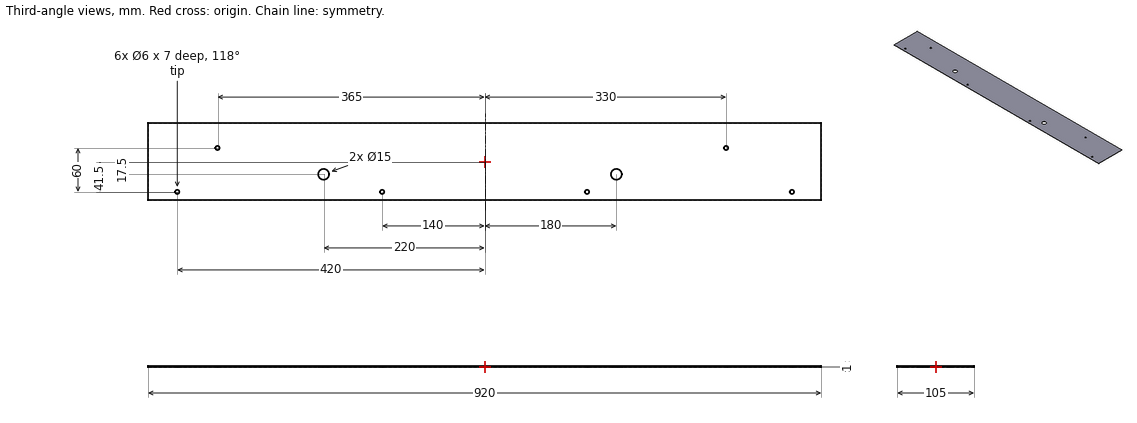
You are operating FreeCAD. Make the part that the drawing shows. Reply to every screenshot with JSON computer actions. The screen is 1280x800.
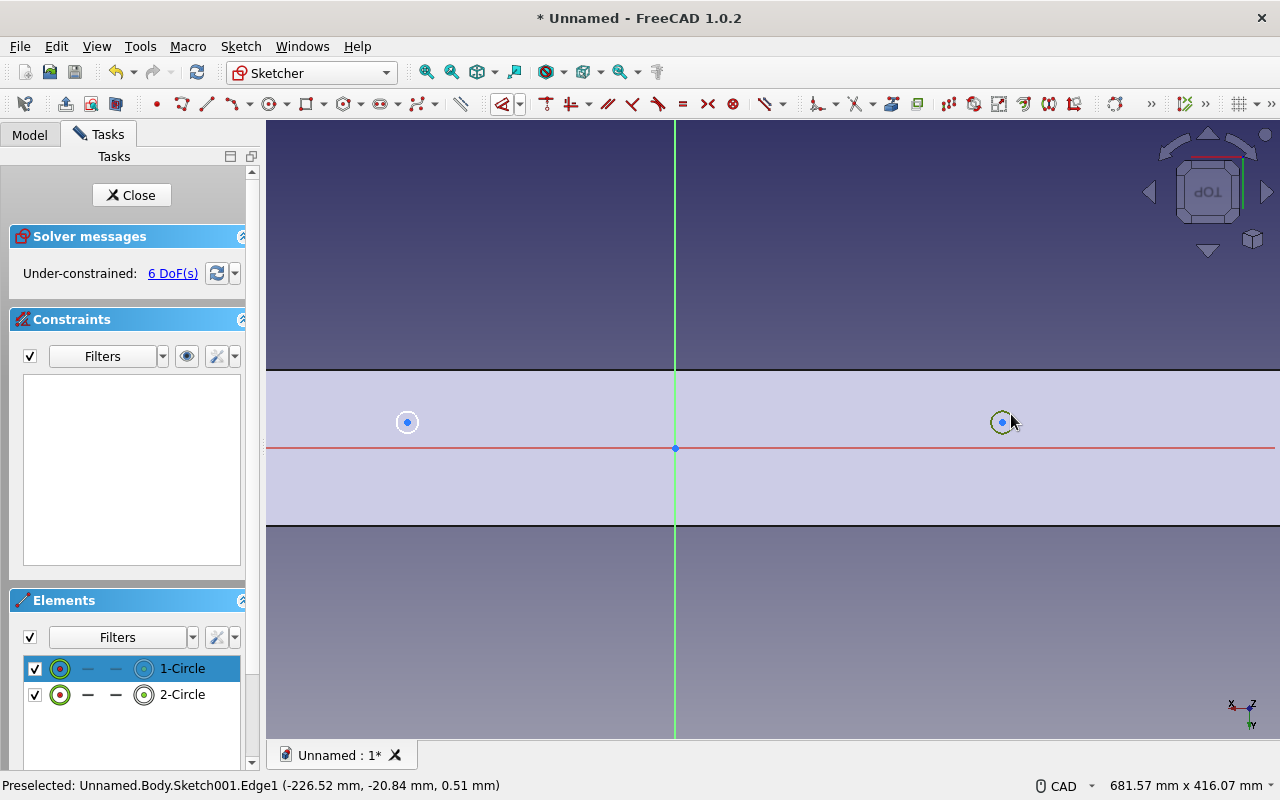
{"action": "scroll", "coordinate": [415, 415], "scroll_direction": "up", "scroll_amount": 2}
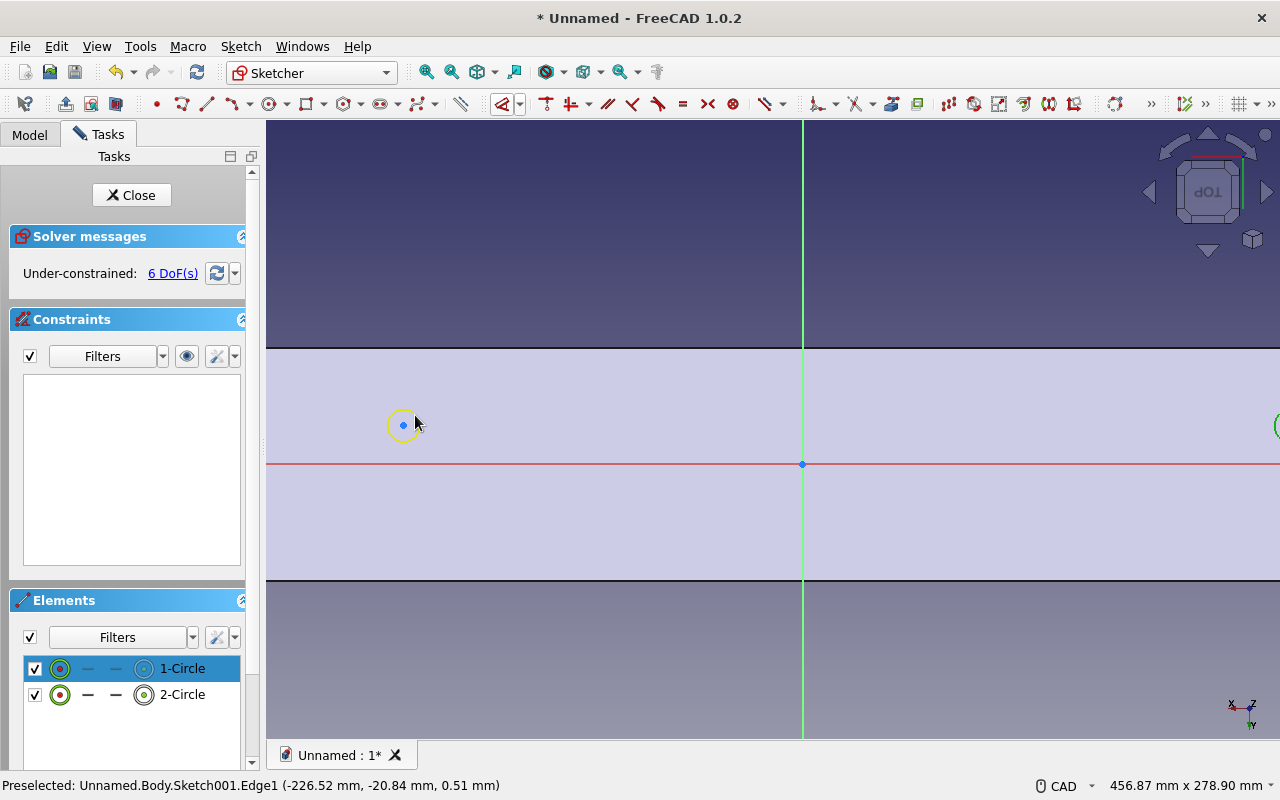
{"action": "left_click", "coordinate": [415, 414]}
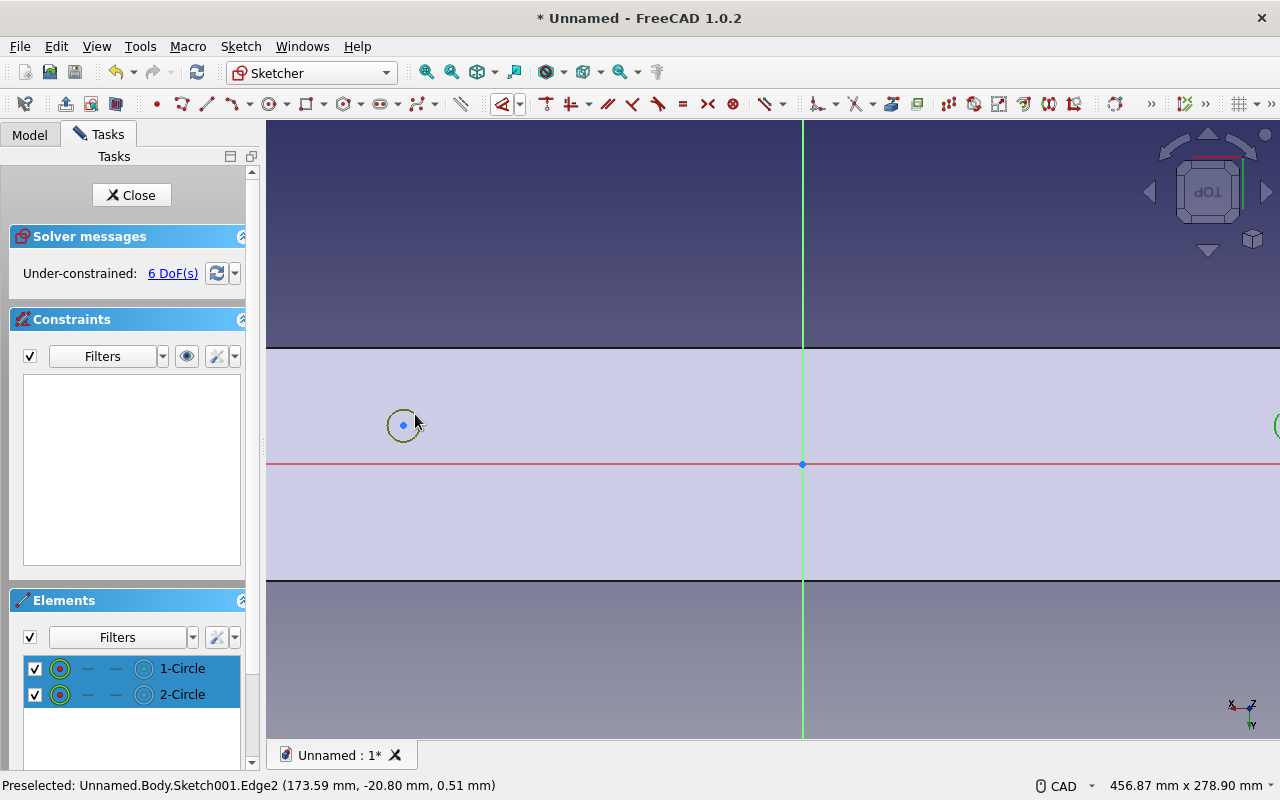
{"action": "left_click", "coordinate": [683, 104]}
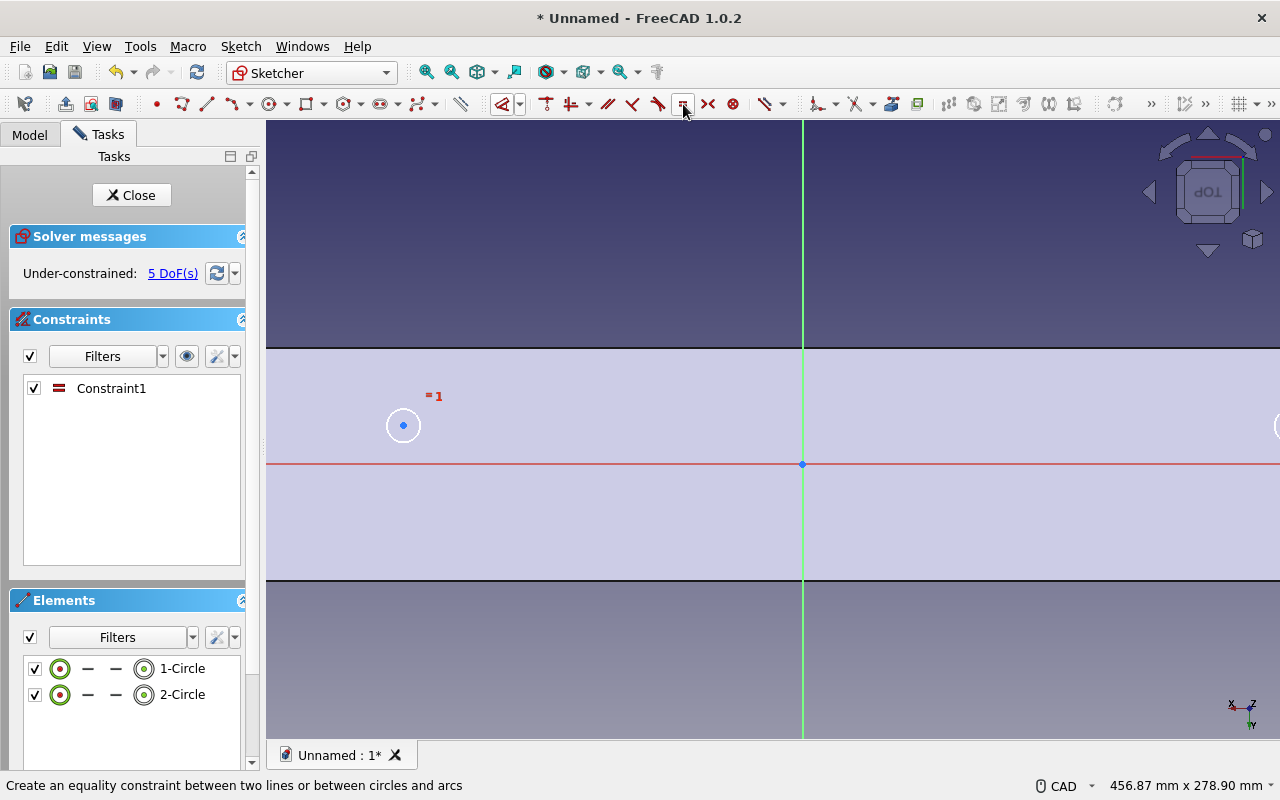
{"action": "scroll", "coordinate": [414, 415], "scroll_direction": "down", "scroll_amount": 2}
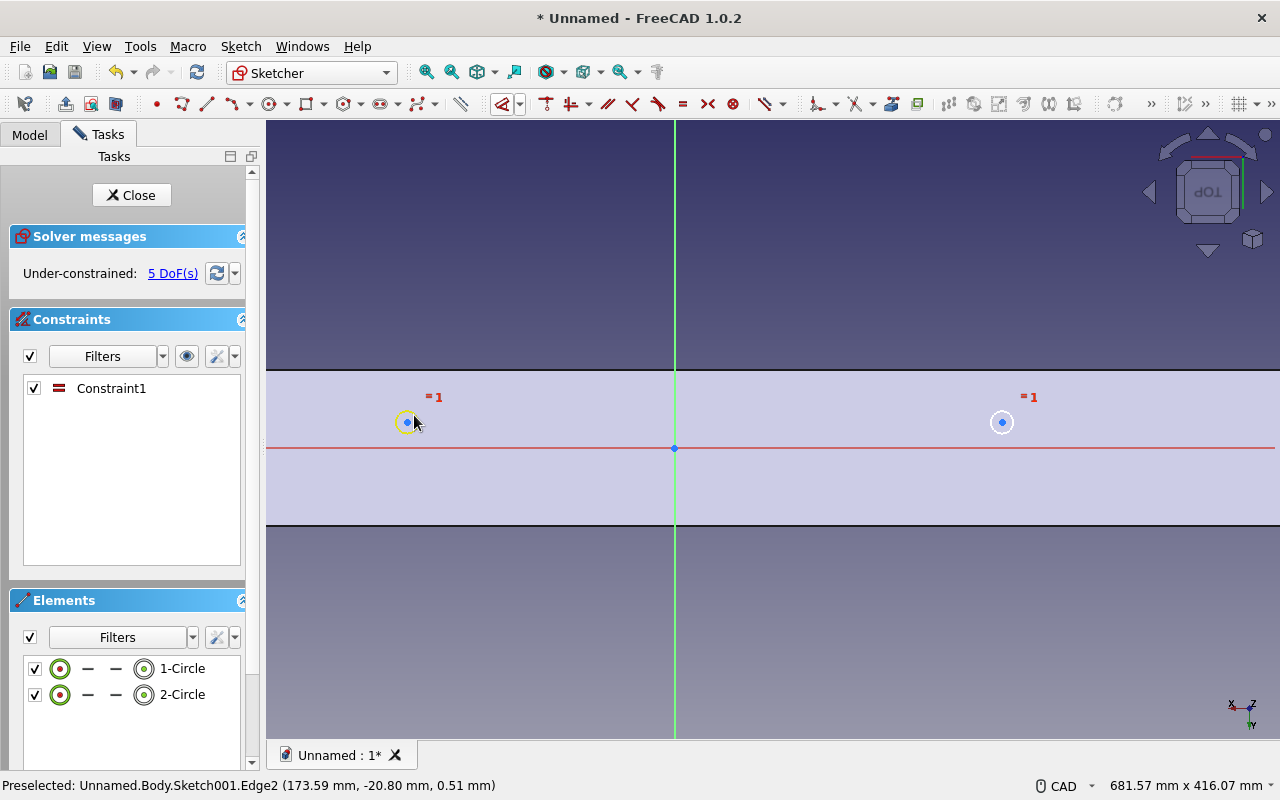
{"action": "scroll", "coordinate": [1010, 415], "scroll_direction": "up", "scroll_amount": 3}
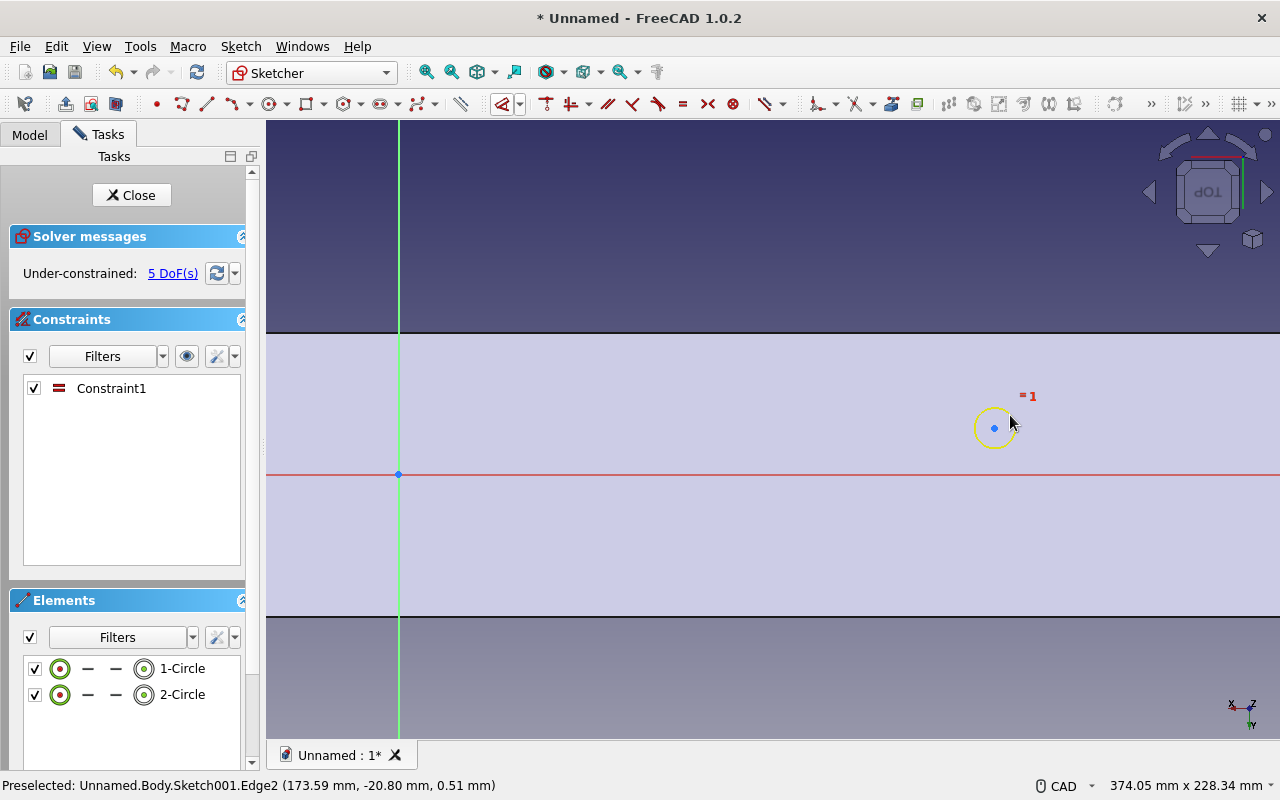
{"action": "left_click", "coordinate": [1009, 414]}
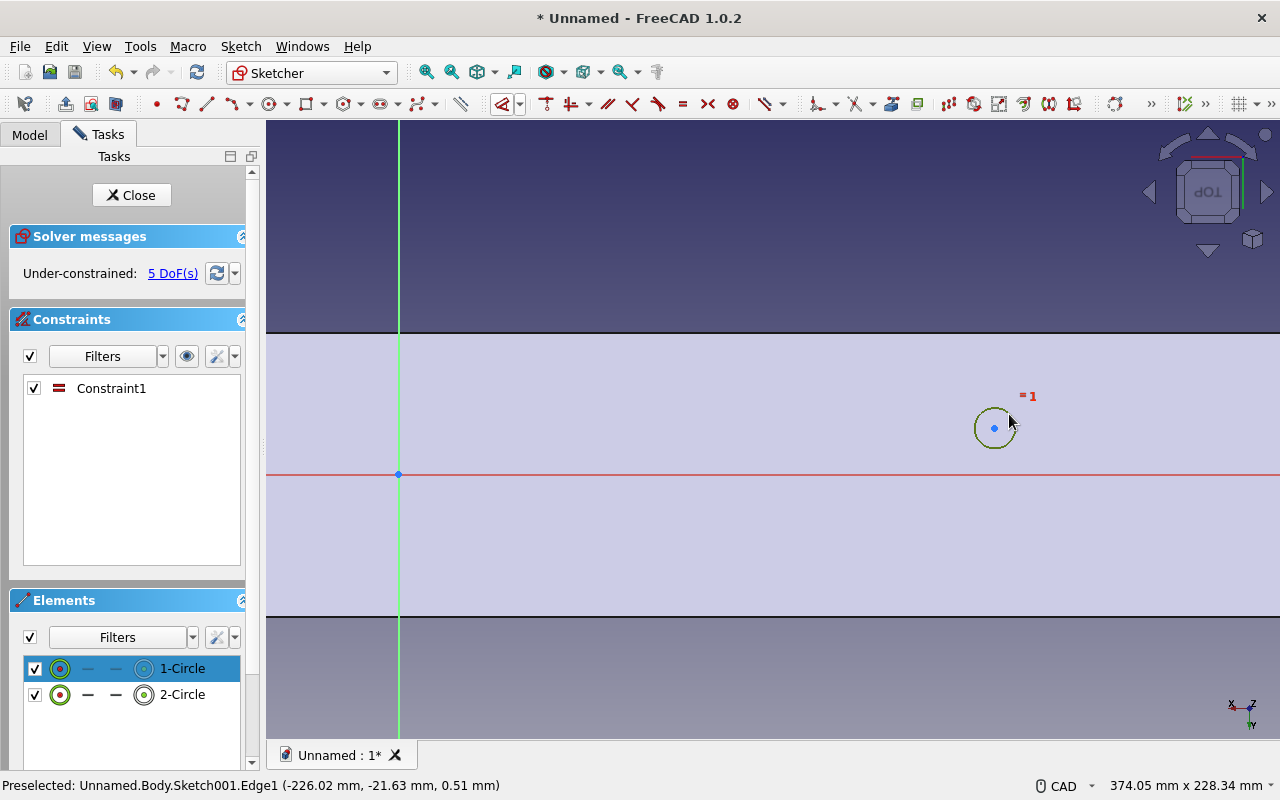
{"action": "key", "text": "k o"}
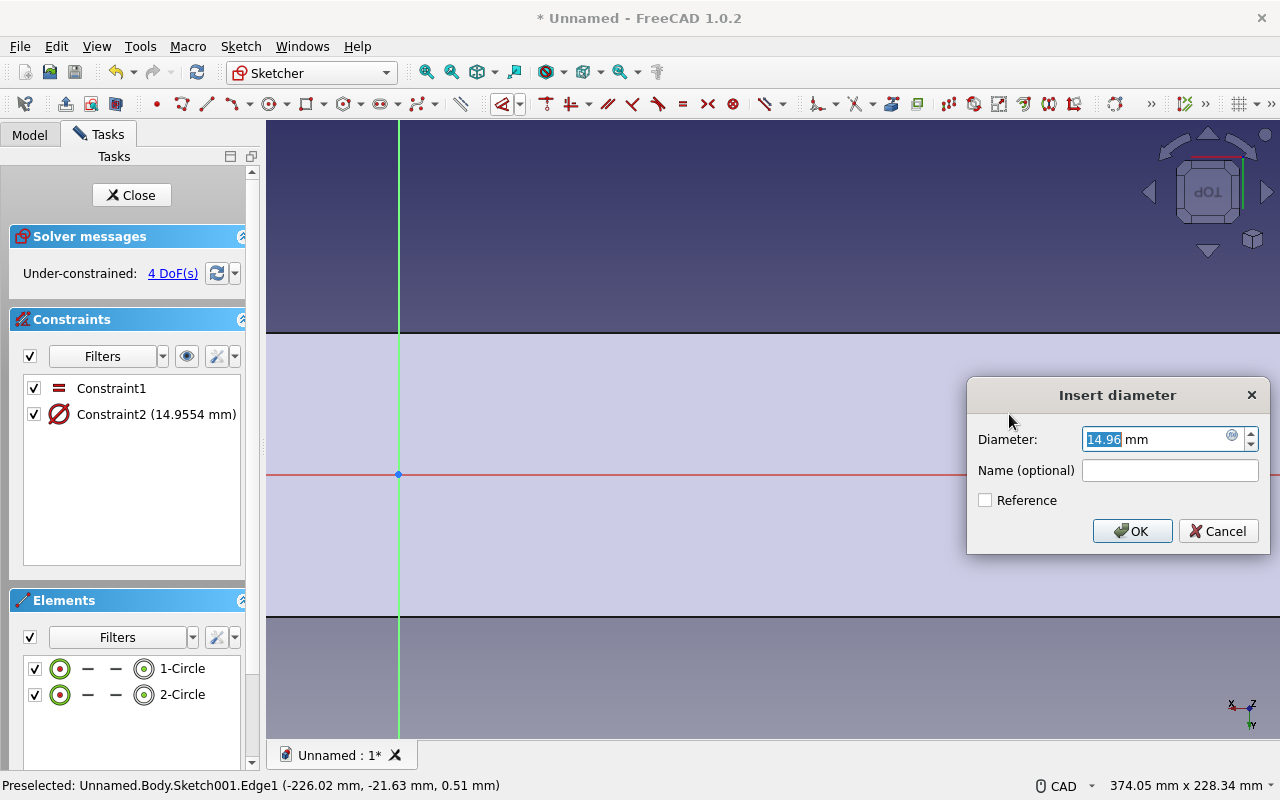
{"action": "type", "text": "15"}
{"action": "key", "text": "Return"}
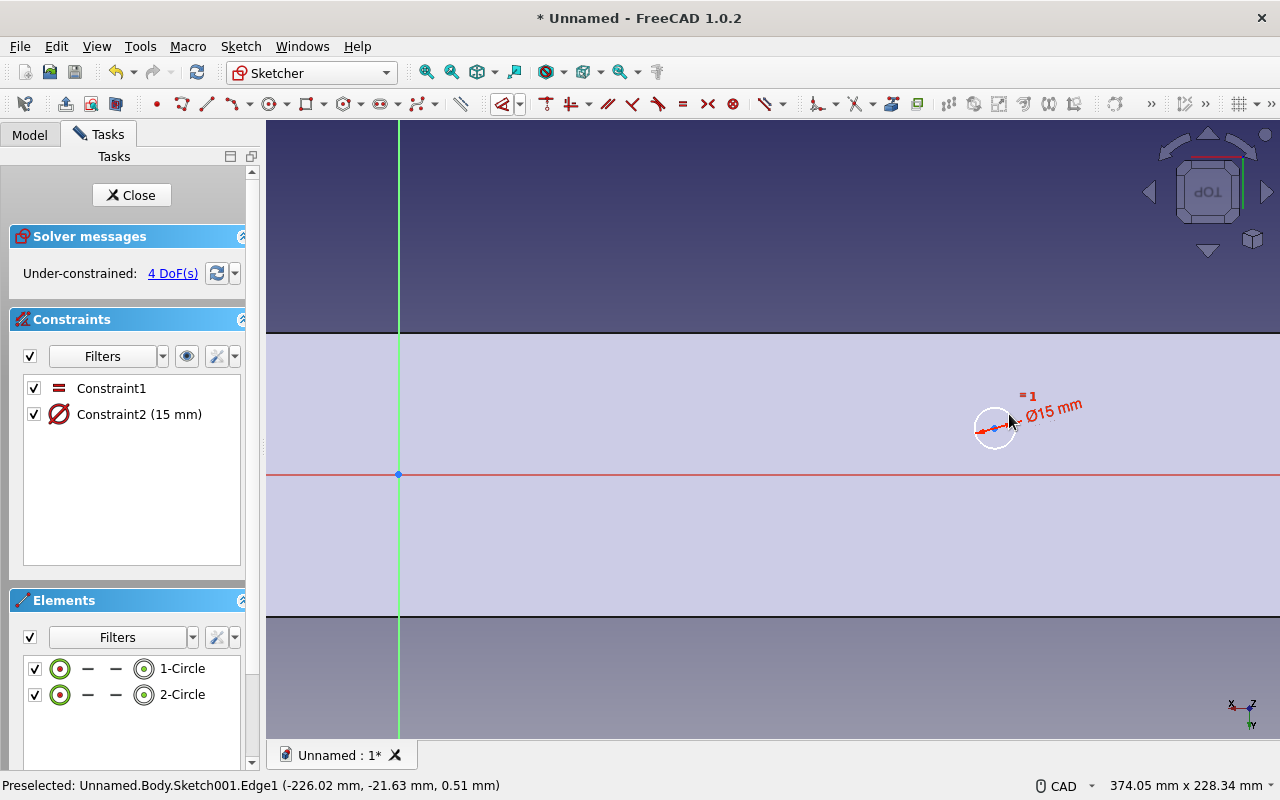
{"action": "left_click", "coordinate": [995, 428]}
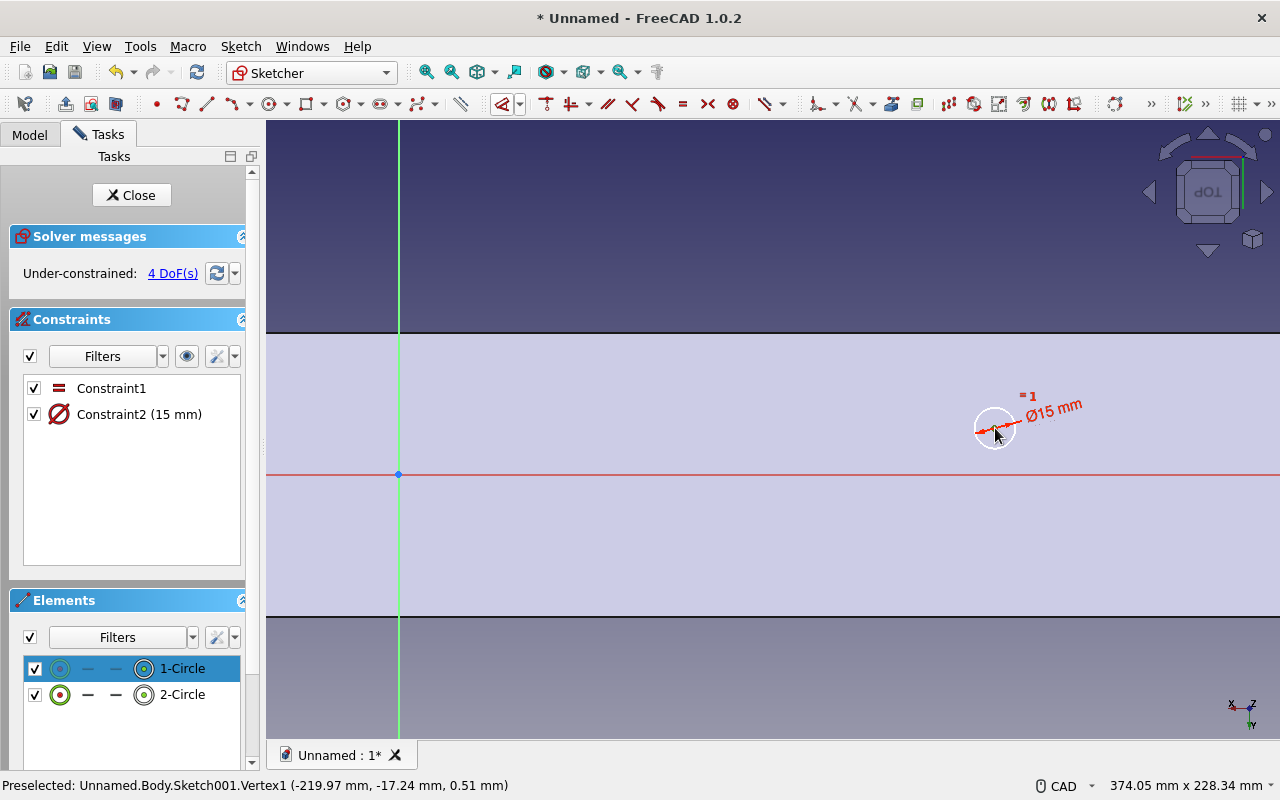
{"action": "left_click", "coordinate": [520, 104]}